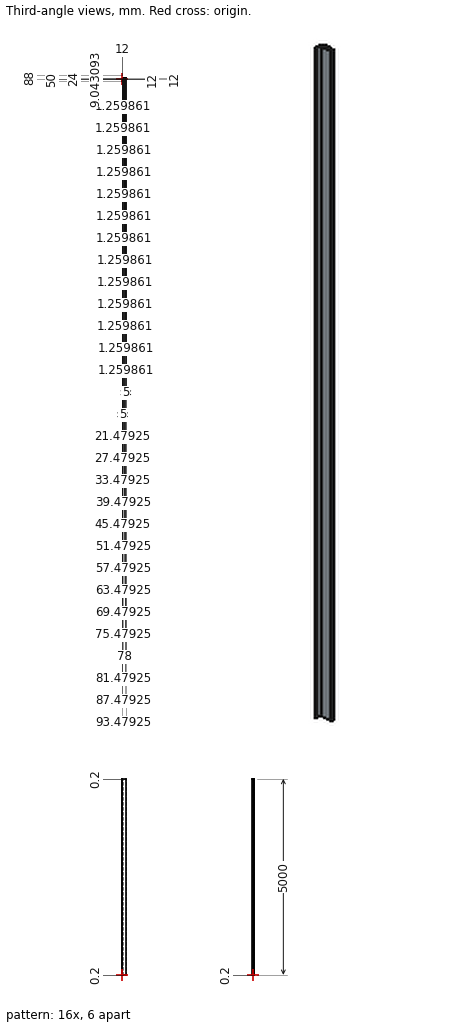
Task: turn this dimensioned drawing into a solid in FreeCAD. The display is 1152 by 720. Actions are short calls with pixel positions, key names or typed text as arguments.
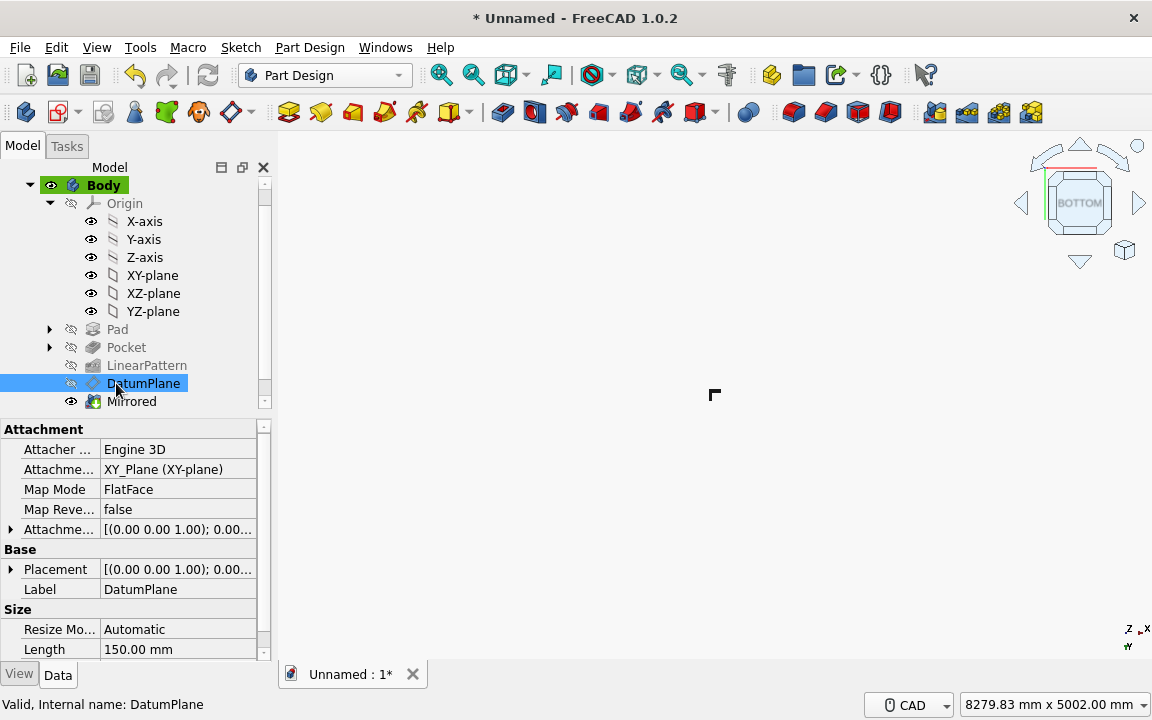
click(442, 76)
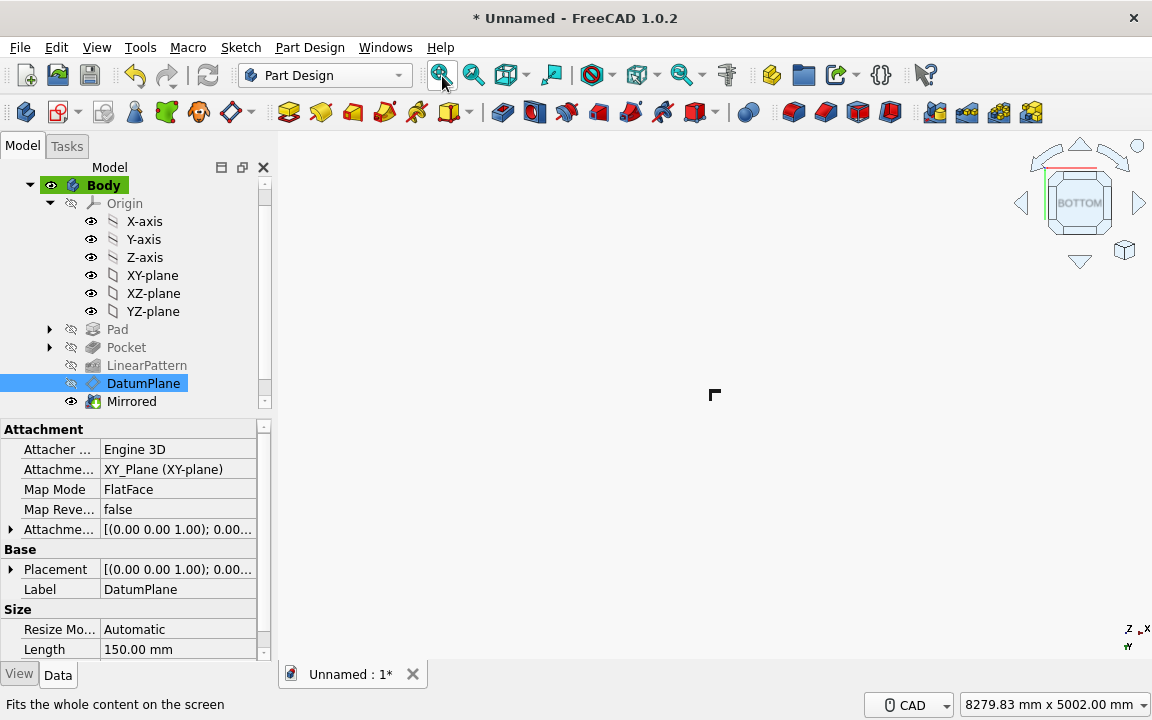
scroll(718, 389, up, 14)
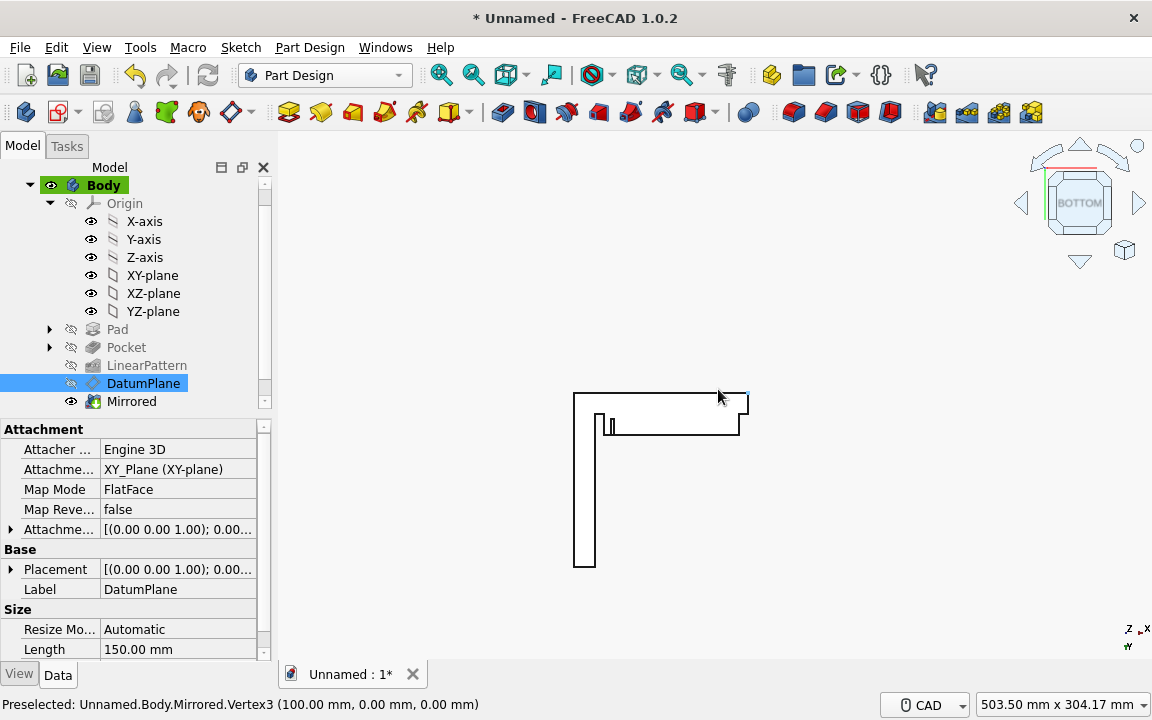
click(710, 405)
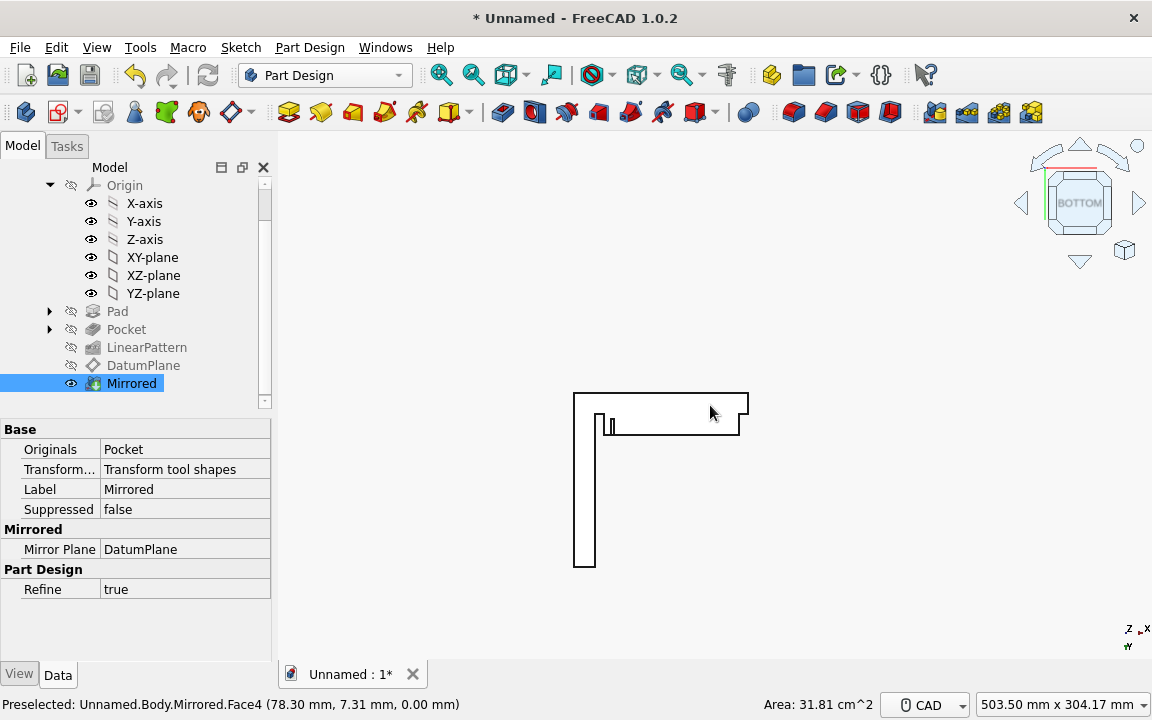
click(58, 112)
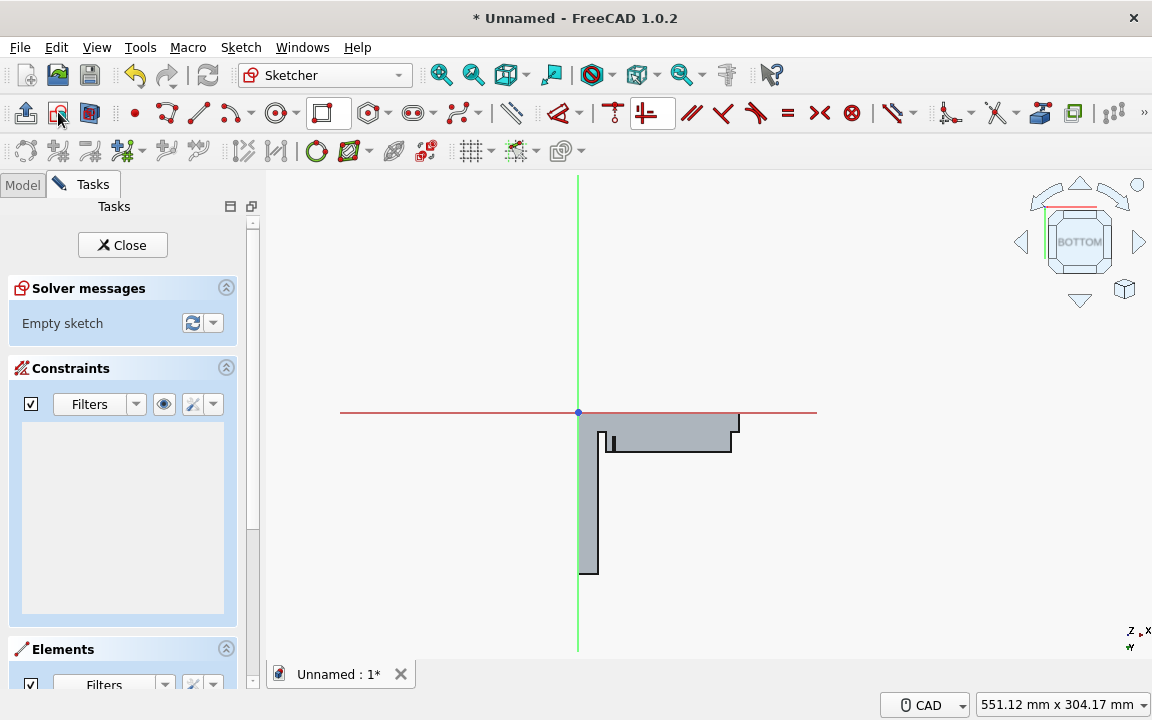
scroll(623, 446, up, 15)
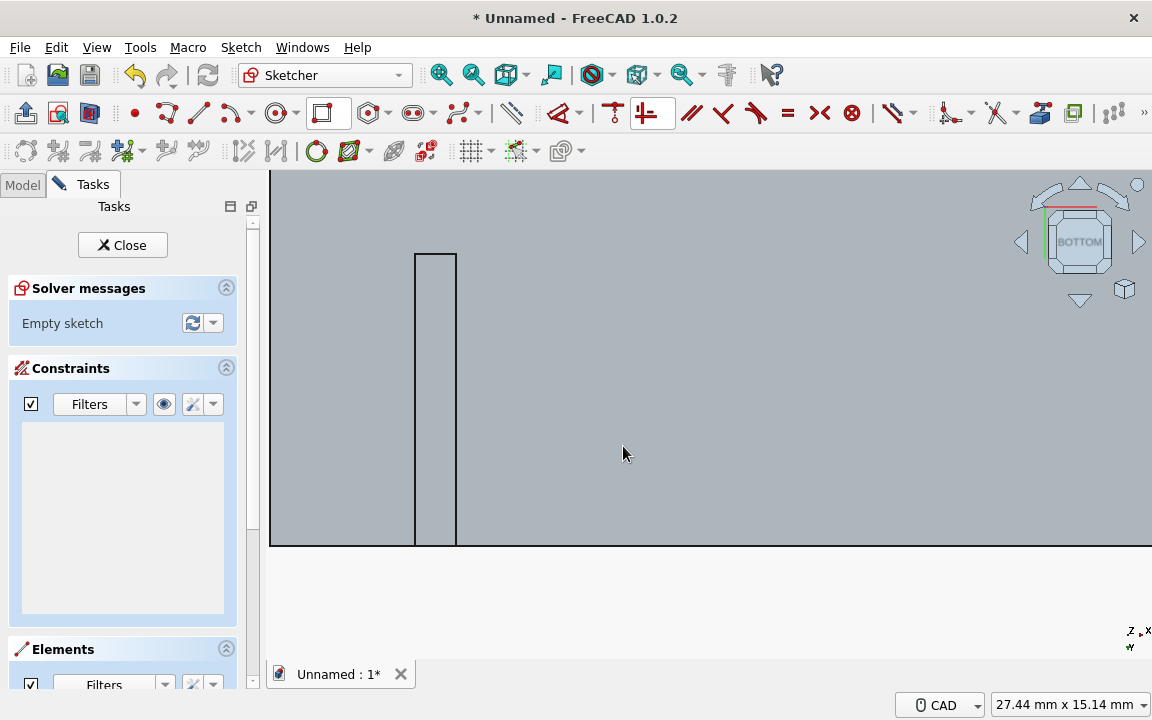
click(322, 114)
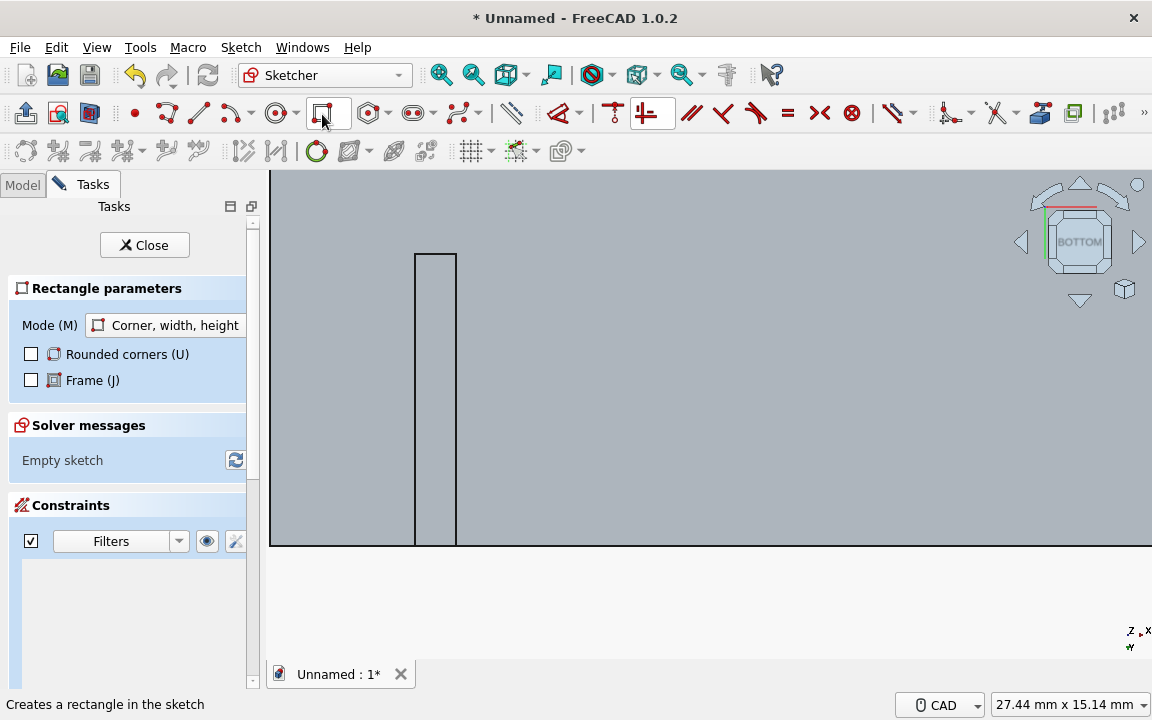
click(609, 254)
click(649, 546)
key(Escape)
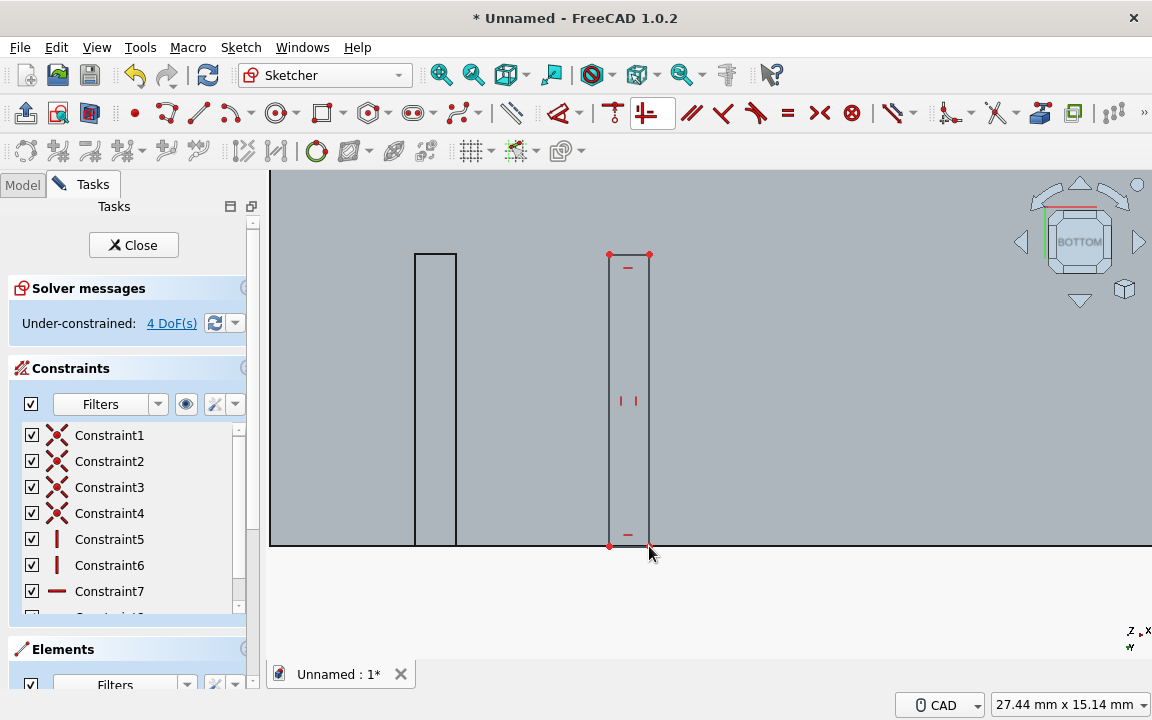
click(558, 114)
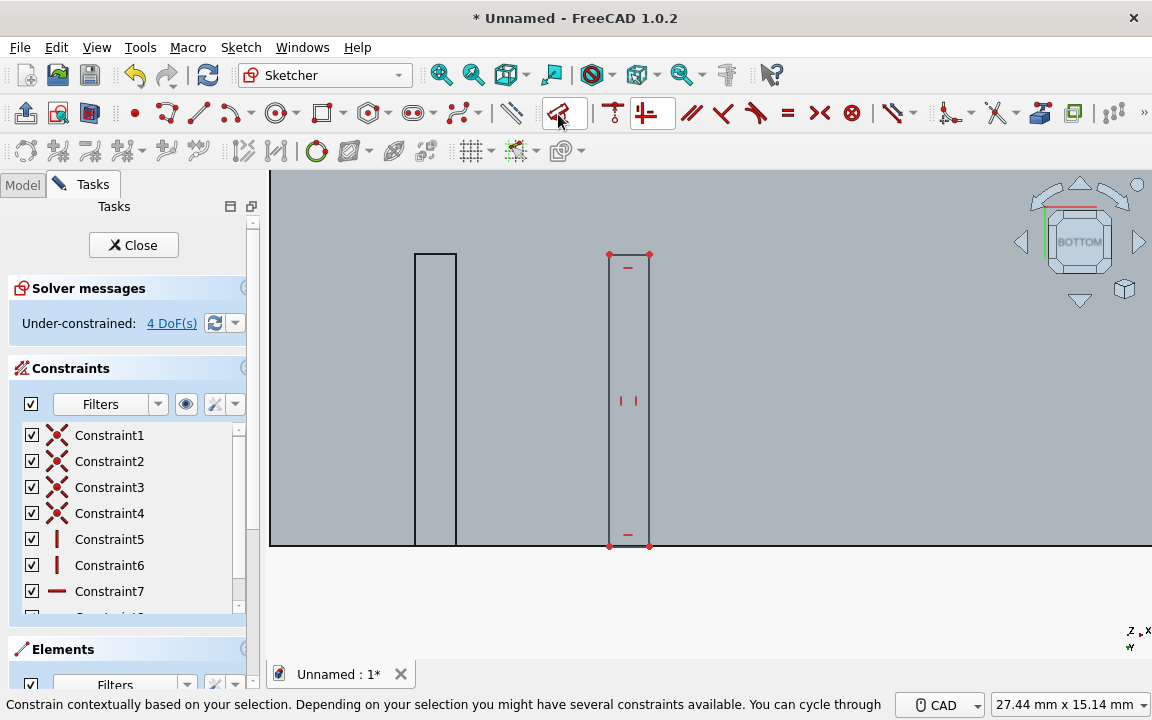
click(609, 547)
click(667, 373)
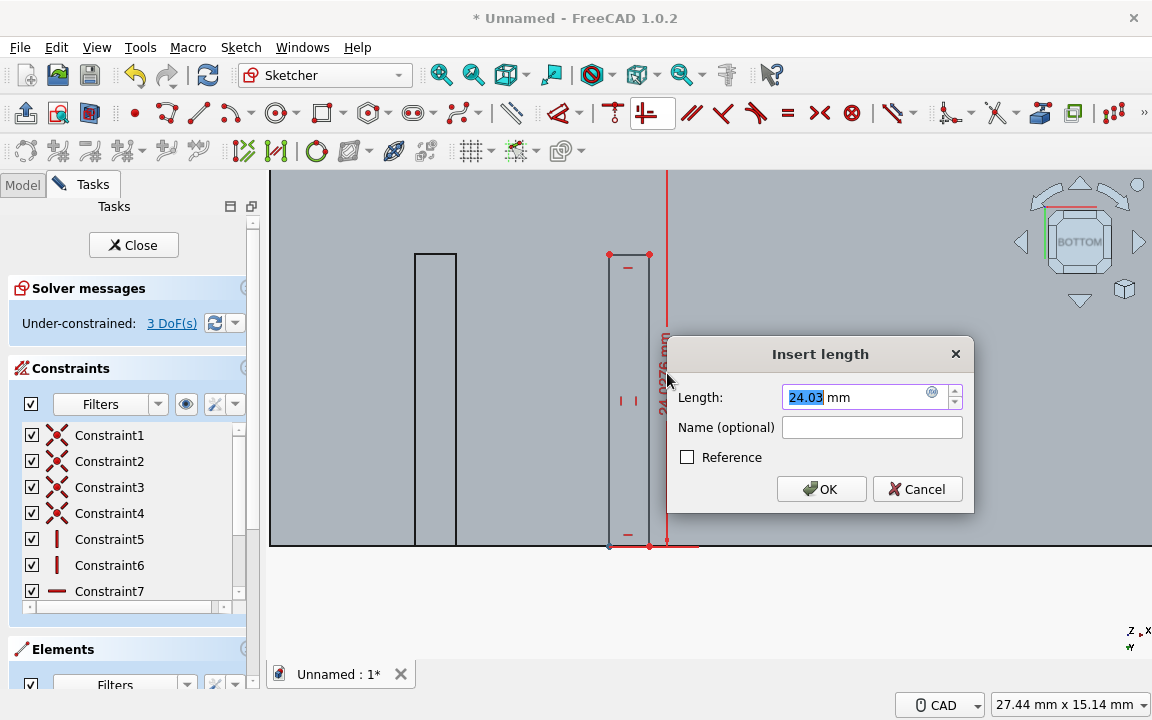
text(24)
key(Return)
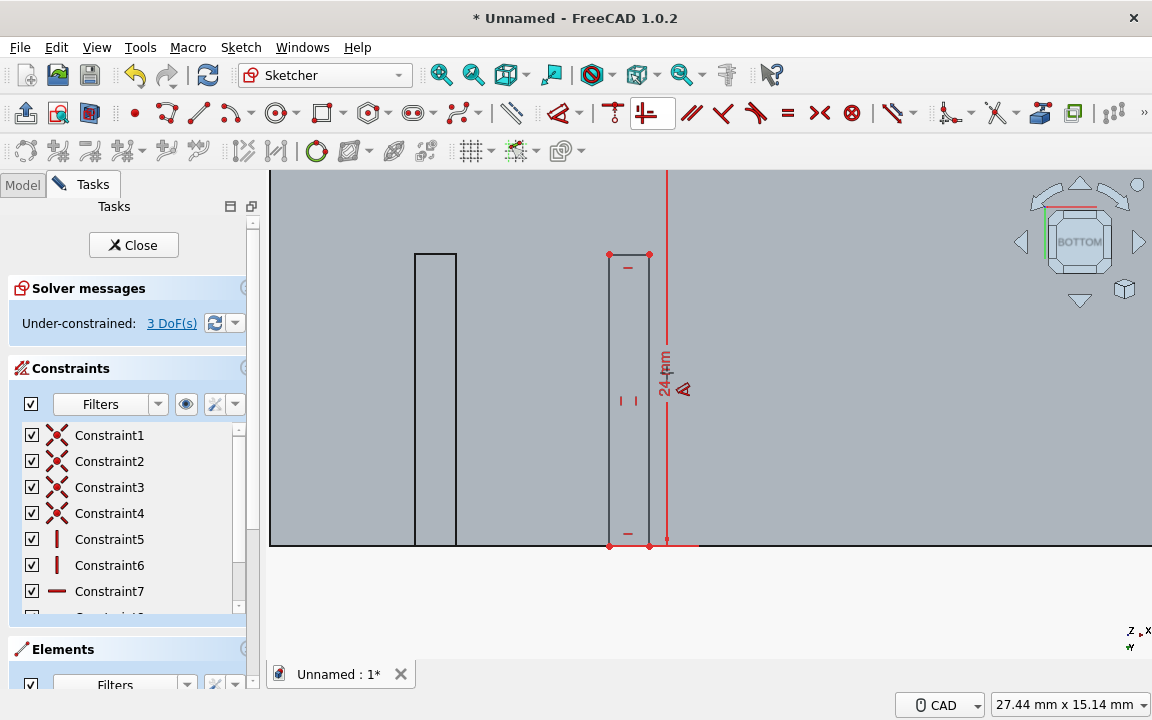
click(609, 342)
click(575, 401)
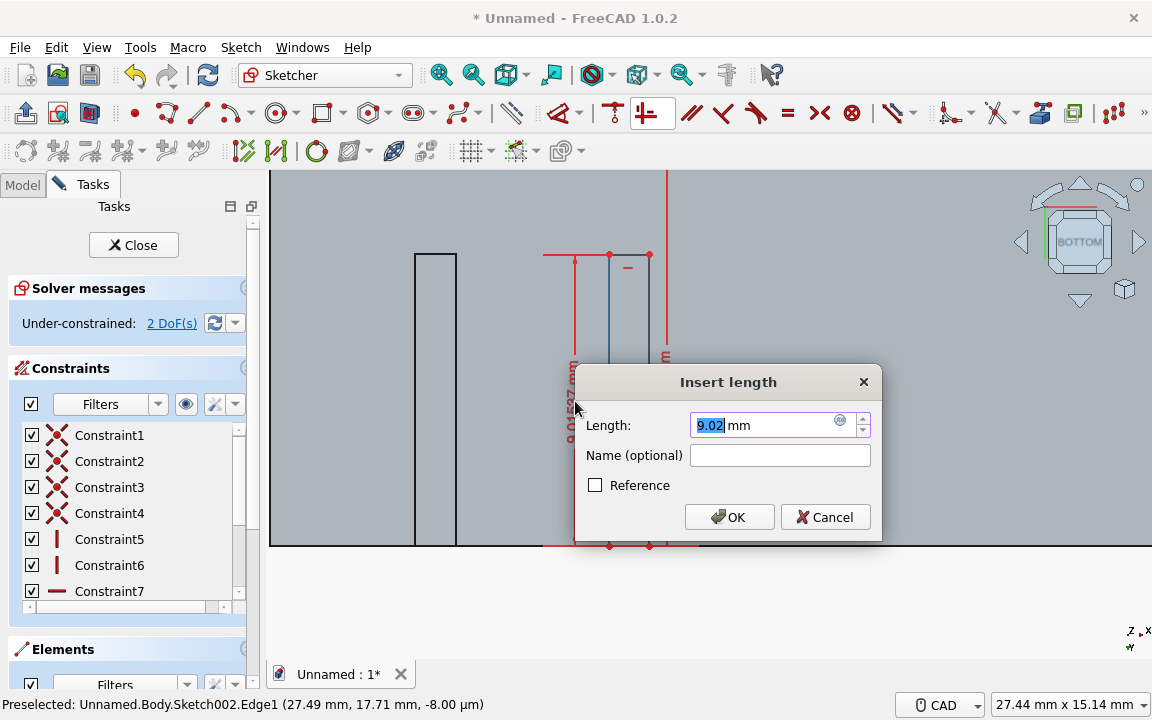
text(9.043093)
key(Return)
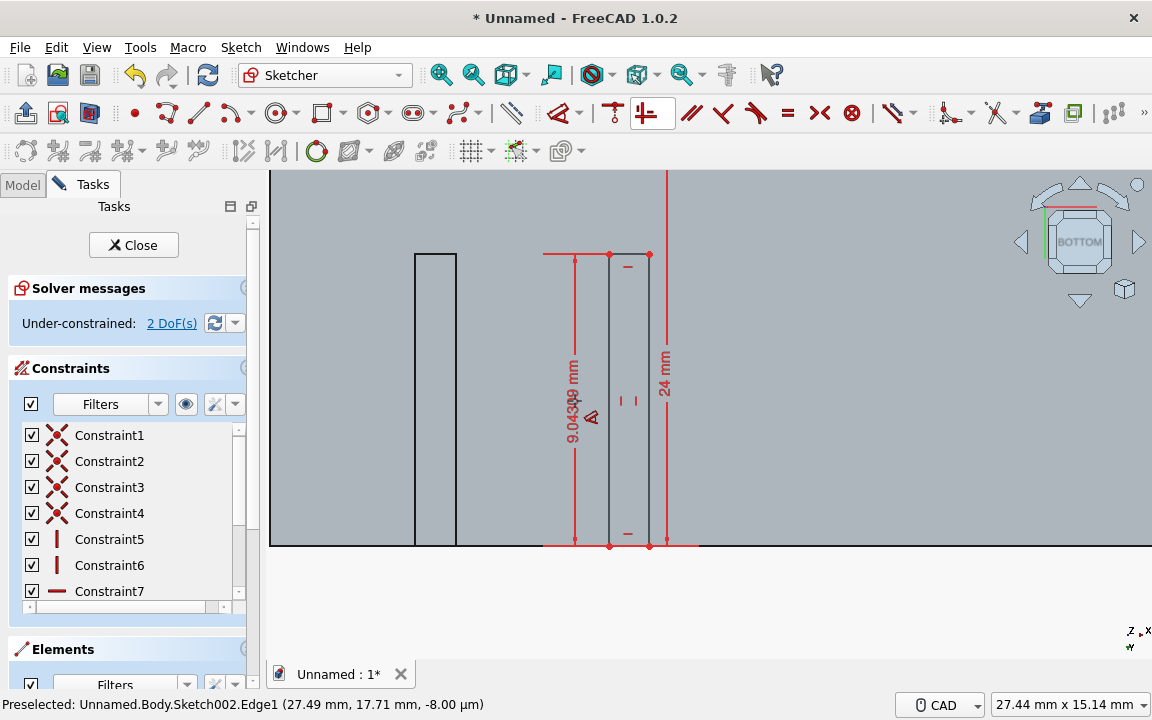
click(621, 546)
click(629, 580)